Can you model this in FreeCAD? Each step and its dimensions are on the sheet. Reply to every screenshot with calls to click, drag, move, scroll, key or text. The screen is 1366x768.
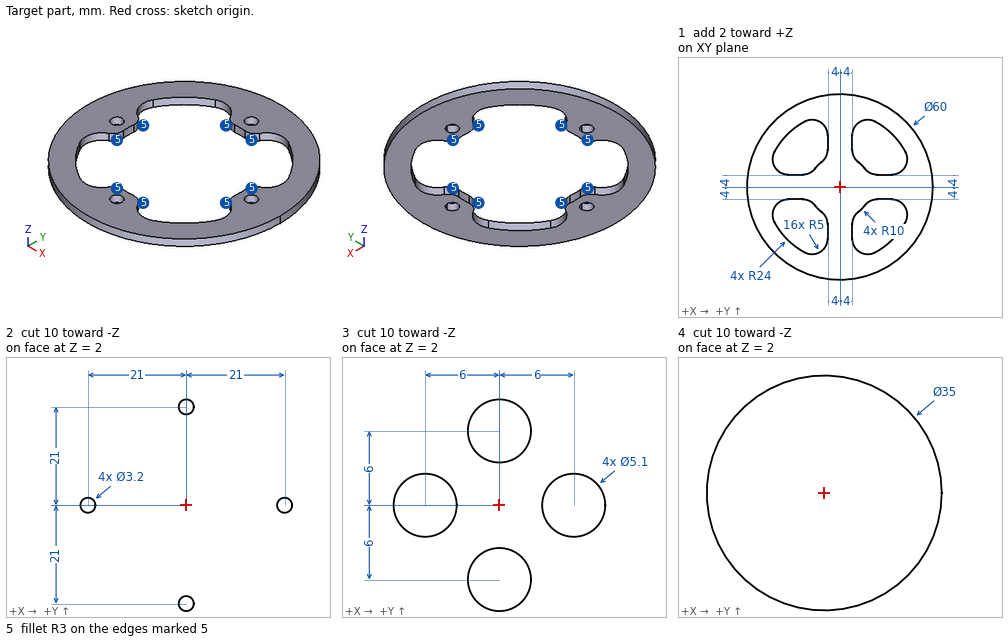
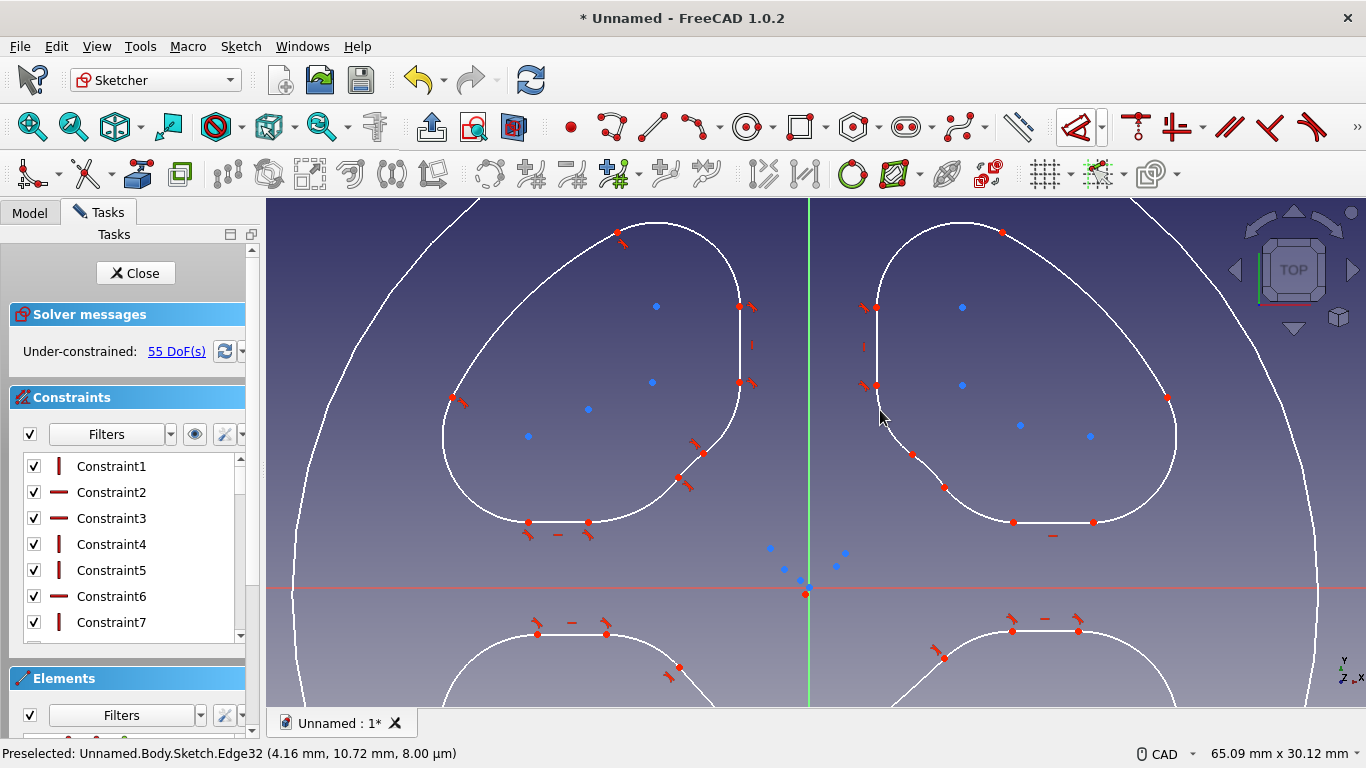
click(1069, 523)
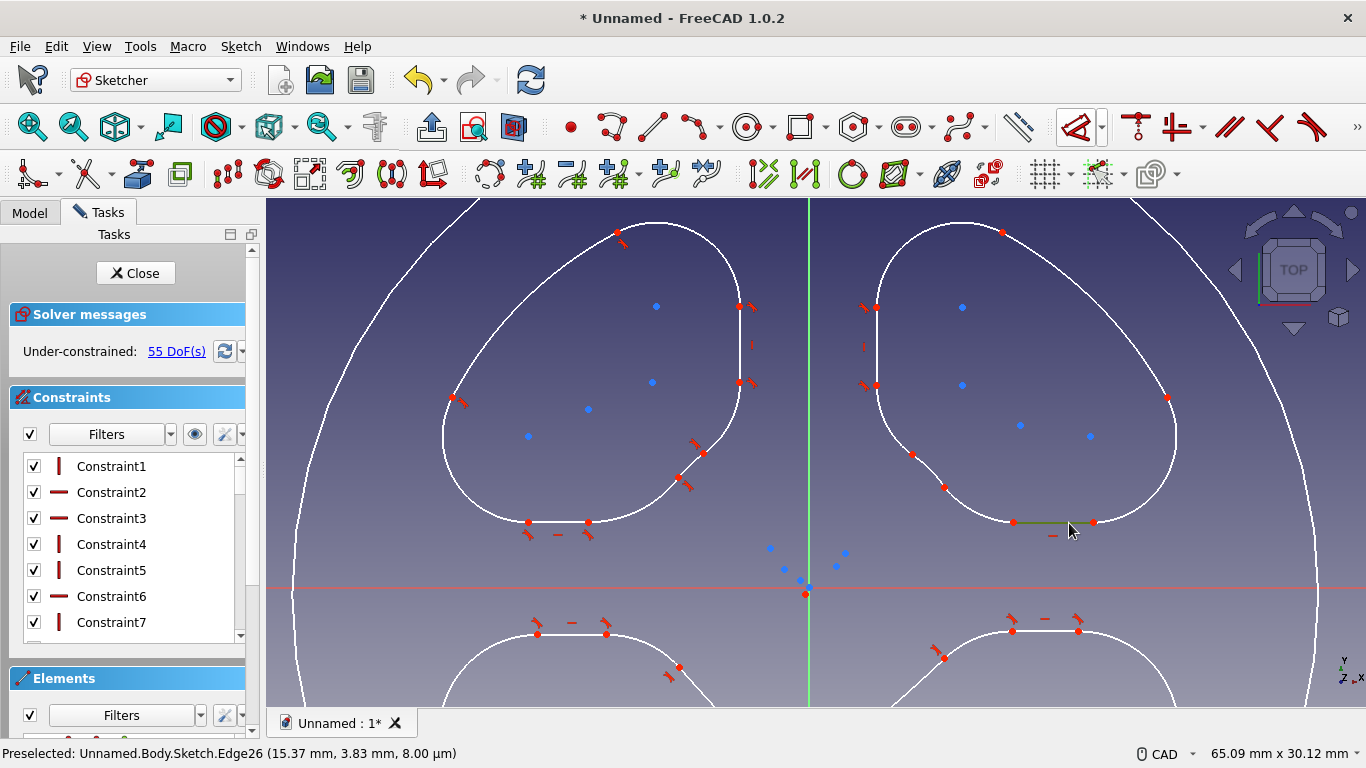
click(1141, 506)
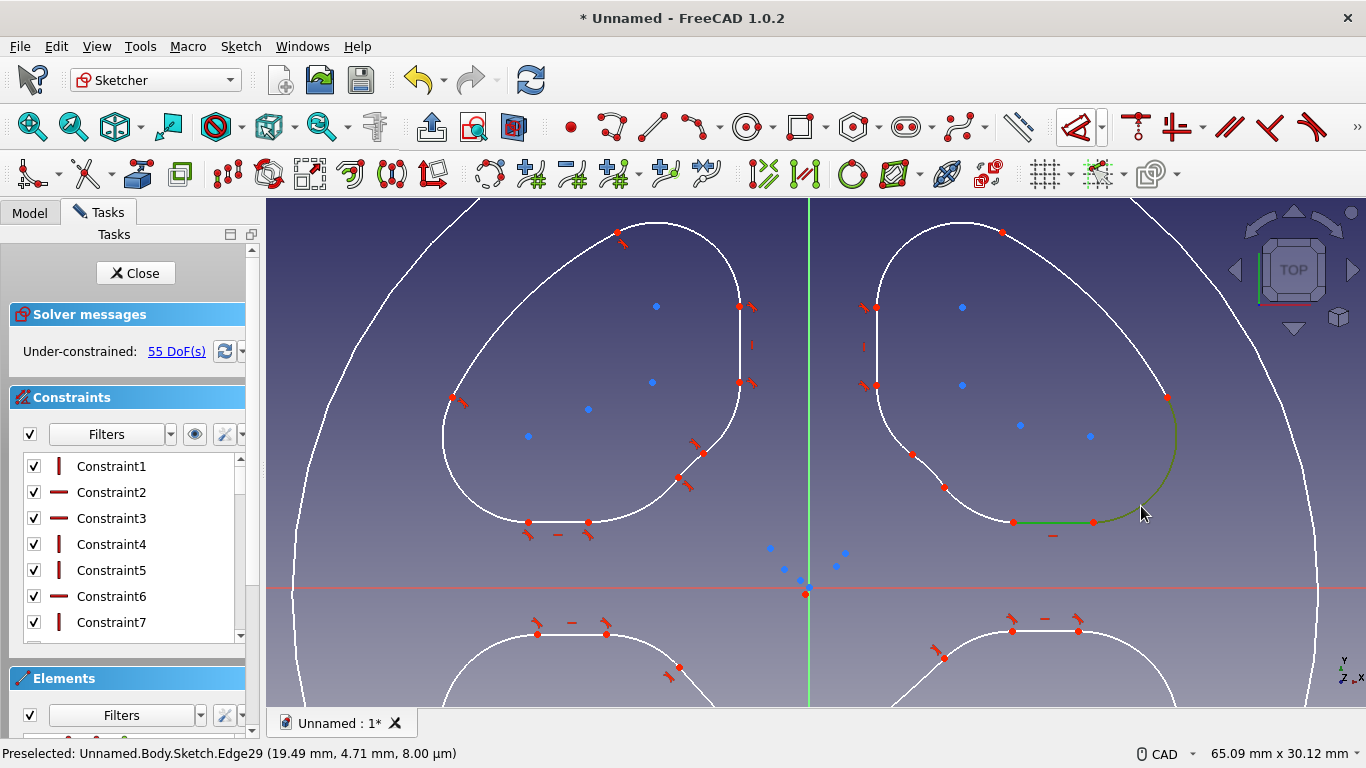
key(t)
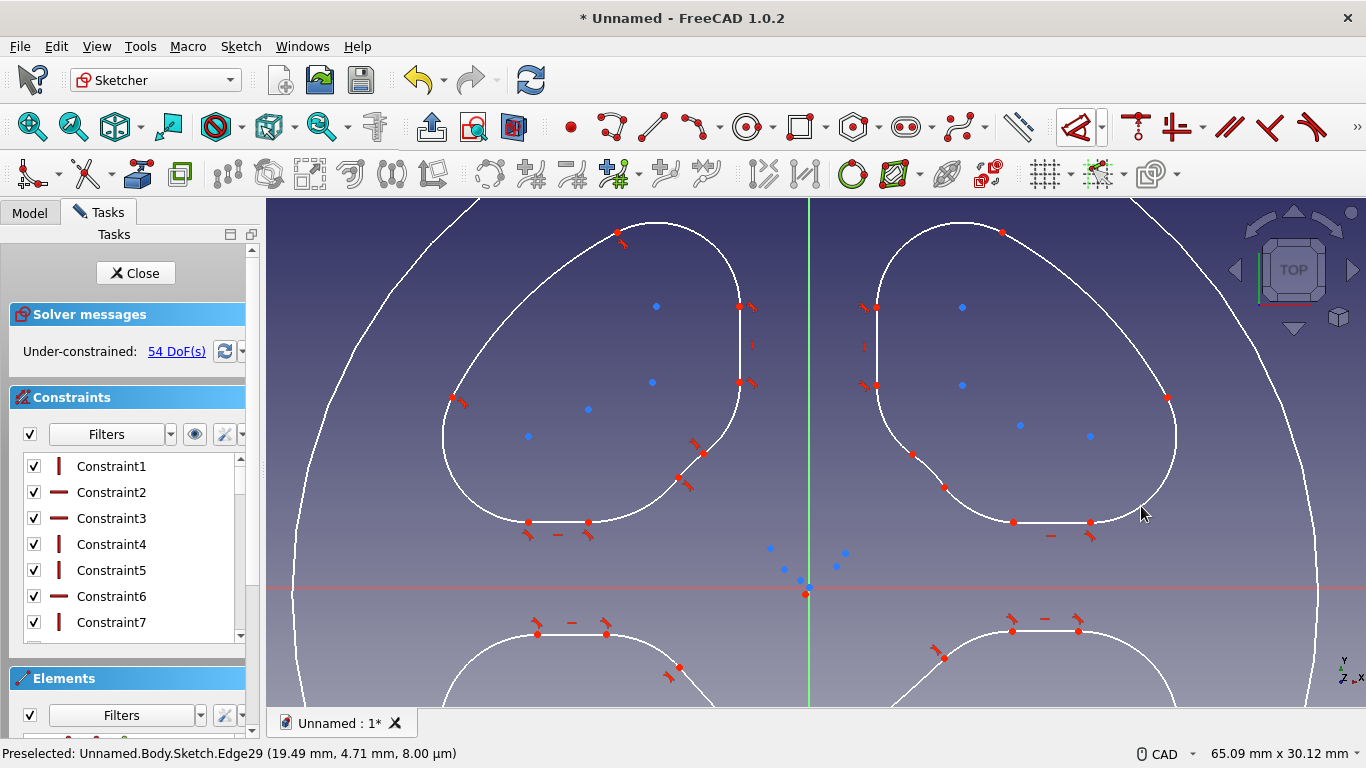
click(1067, 523)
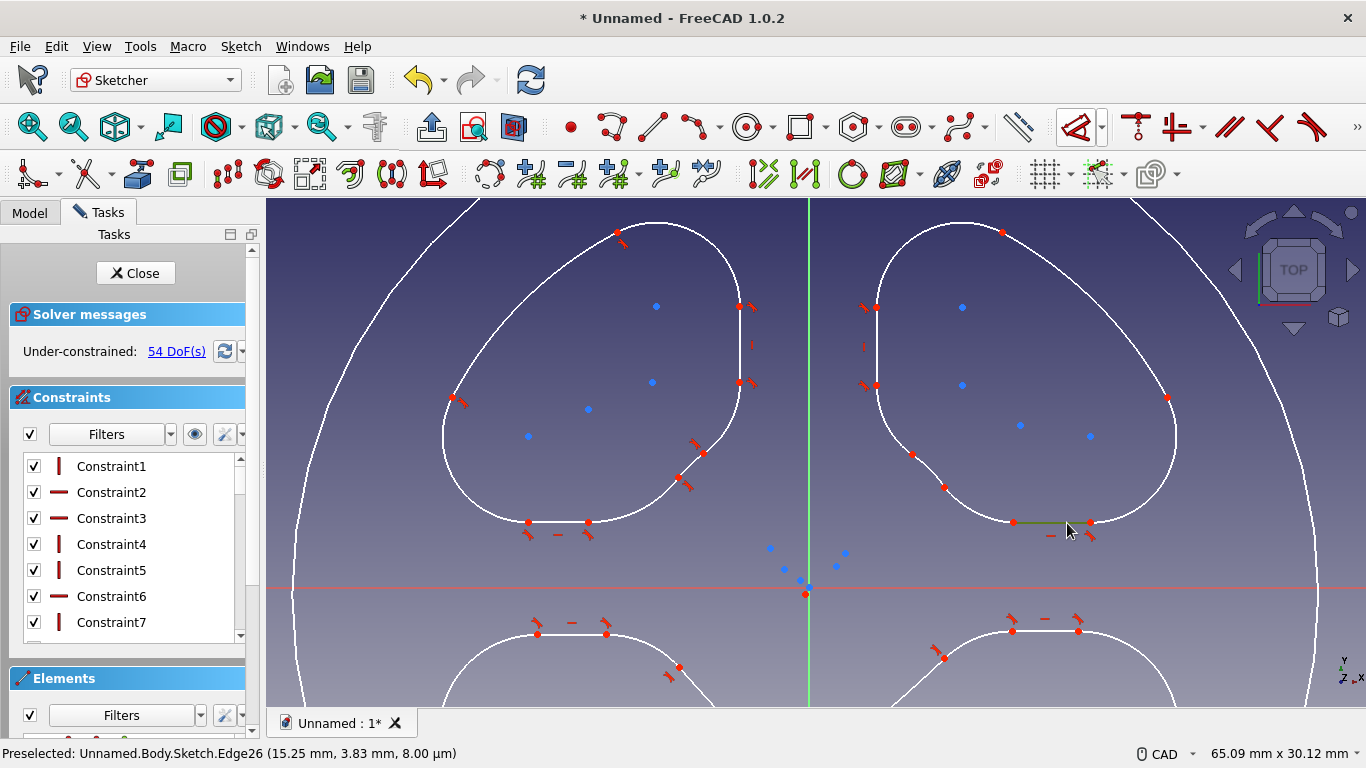
click(962, 504)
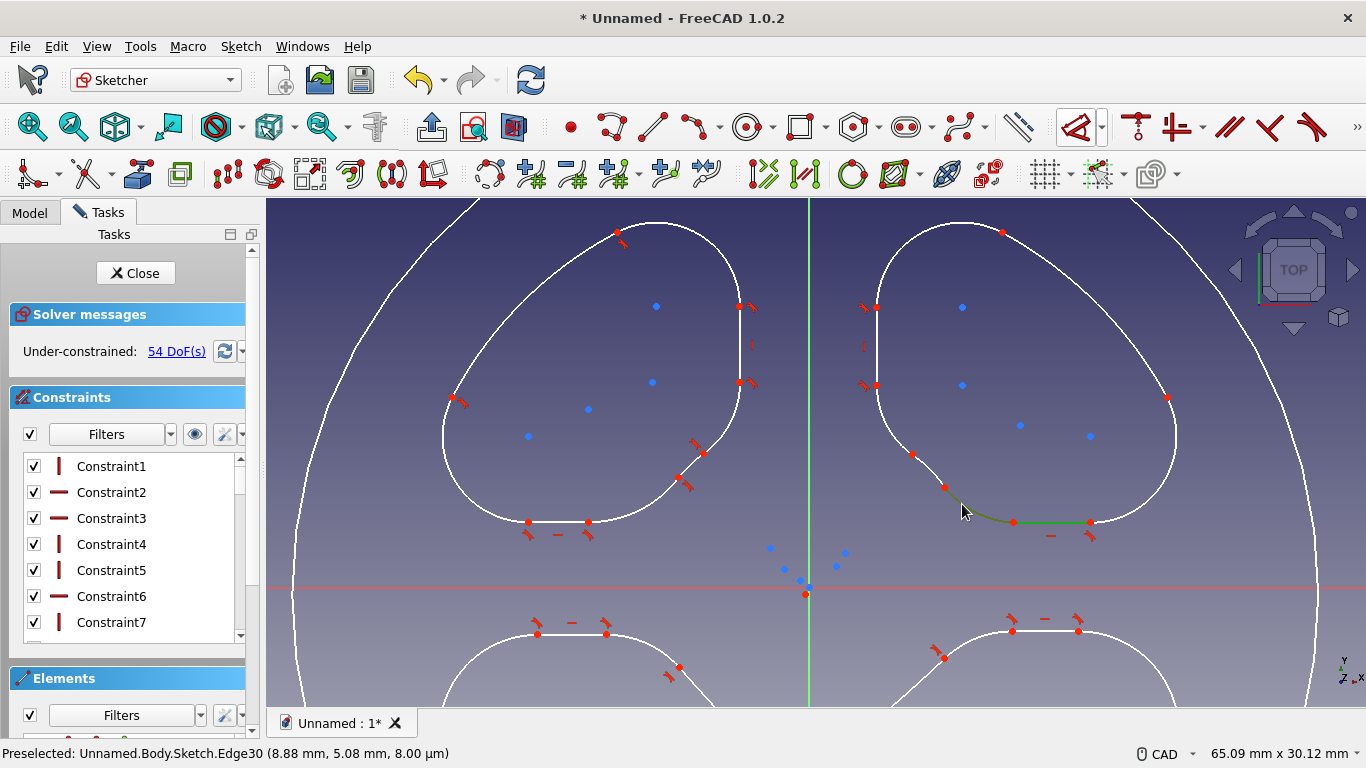
key(t)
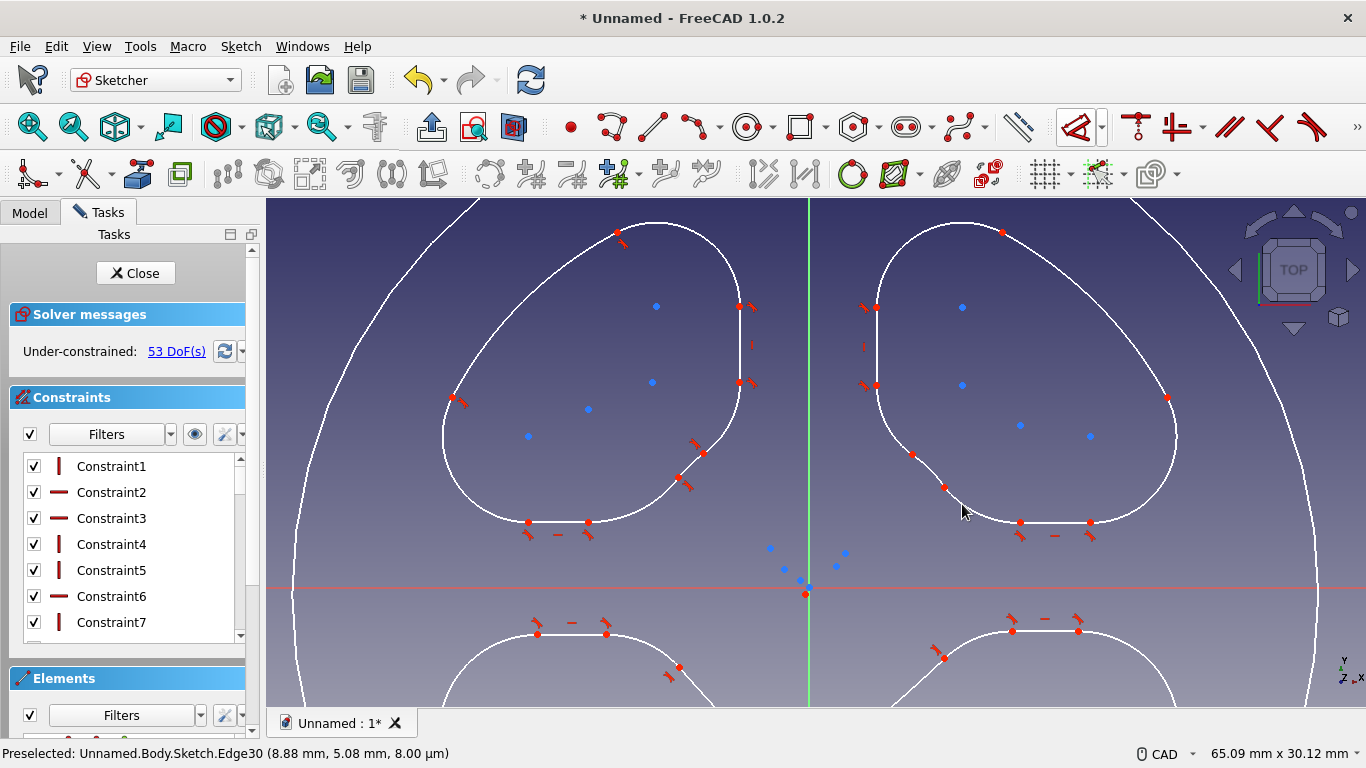
click(893, 258)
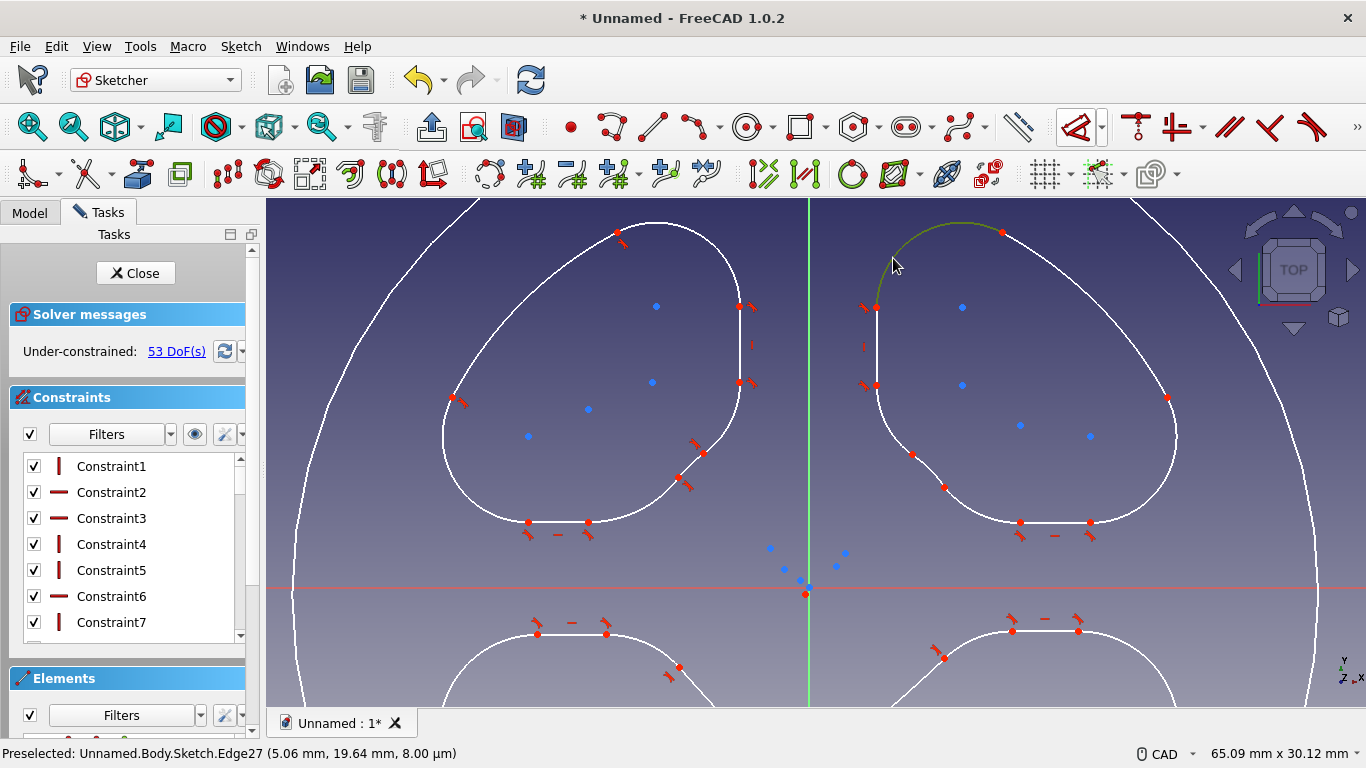
click(1128, 339)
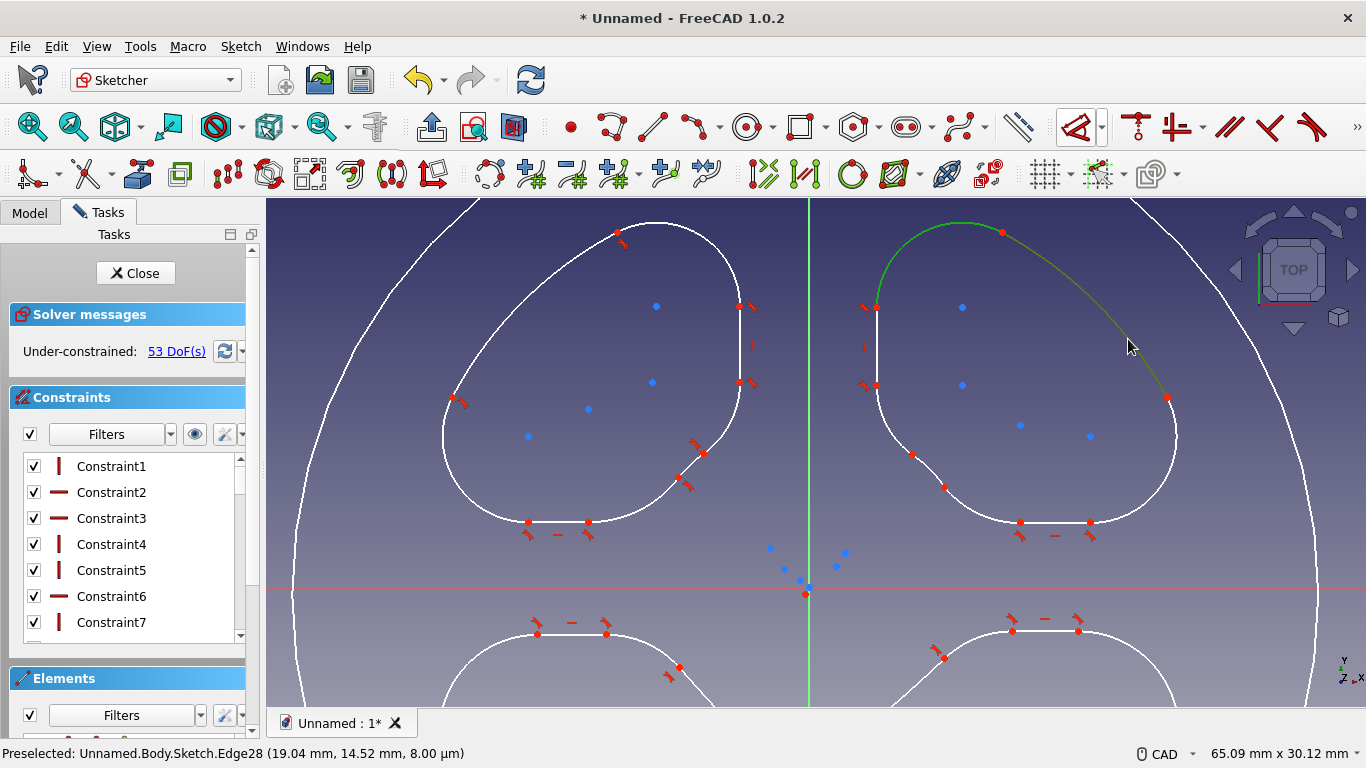
key(t)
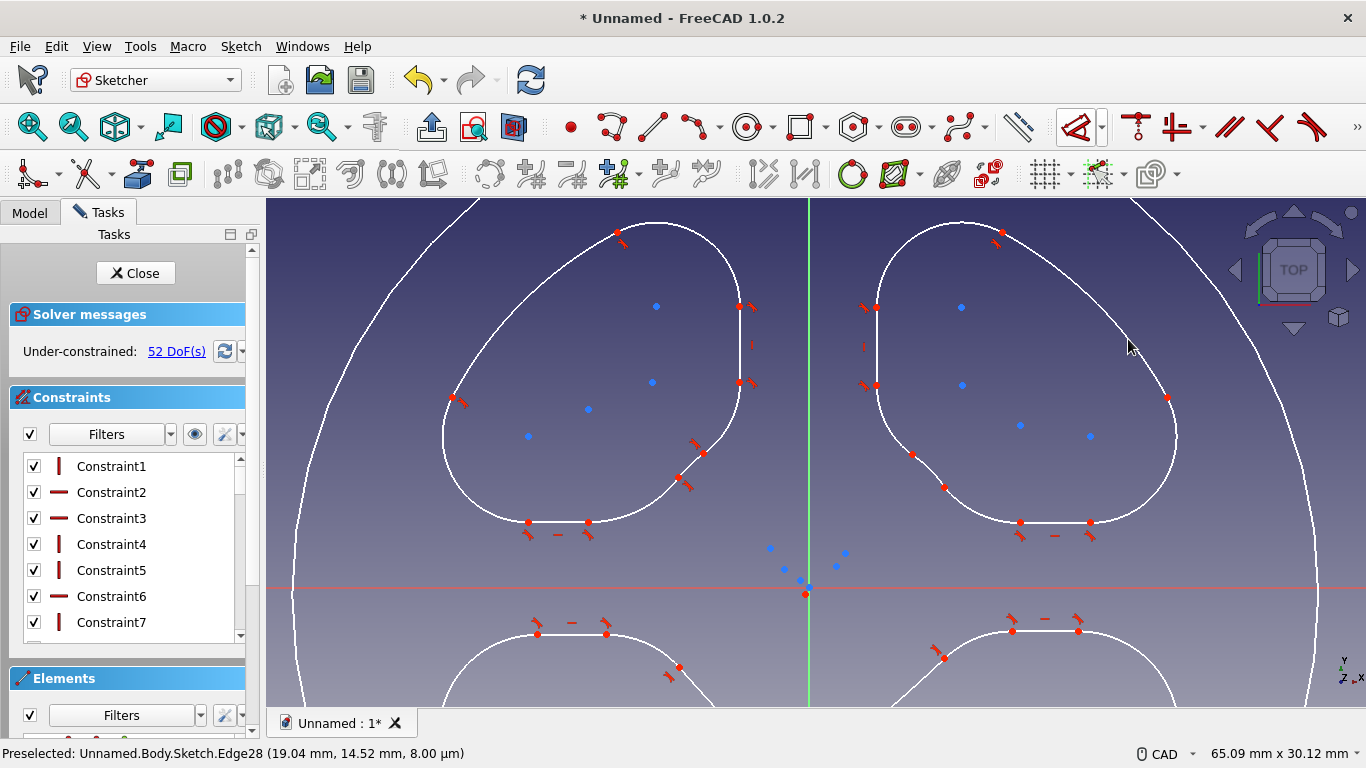
click(1128, 339)